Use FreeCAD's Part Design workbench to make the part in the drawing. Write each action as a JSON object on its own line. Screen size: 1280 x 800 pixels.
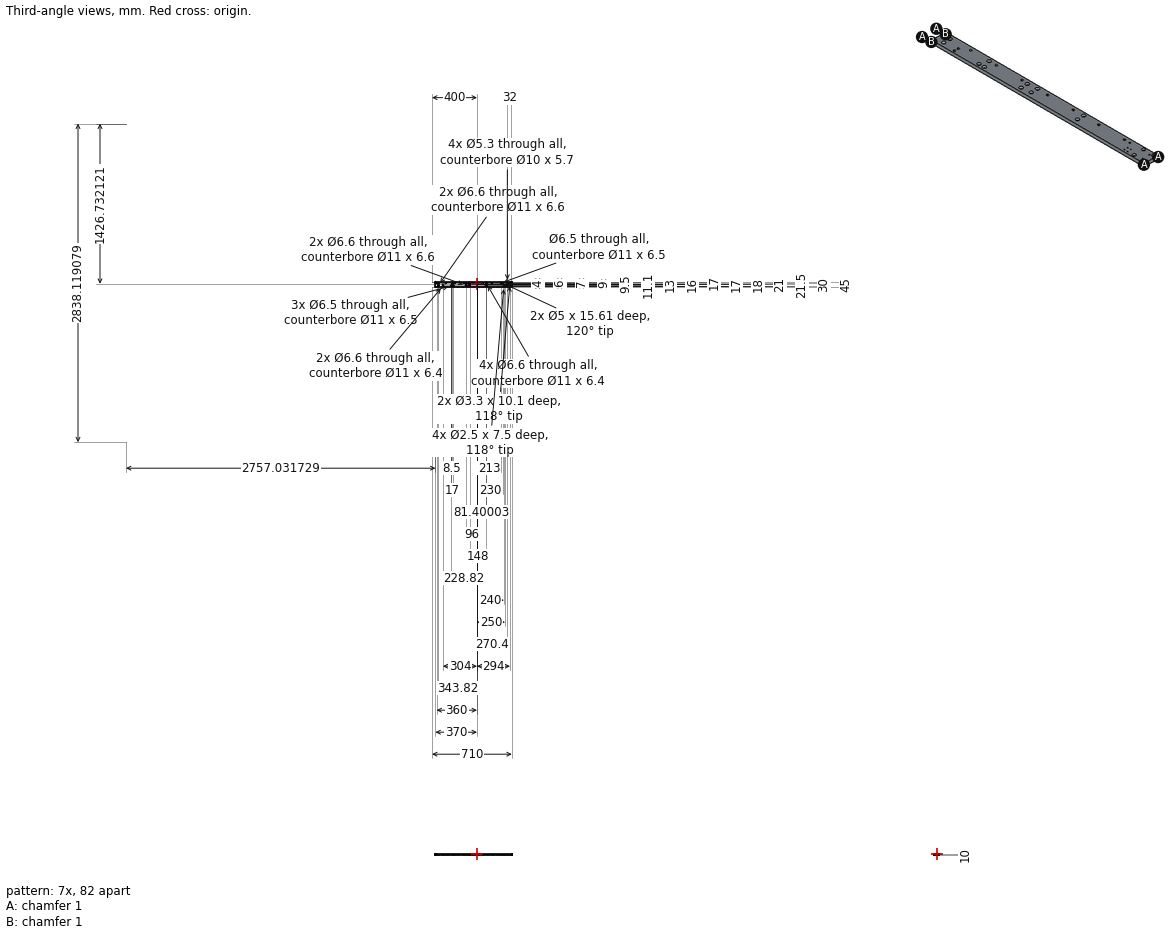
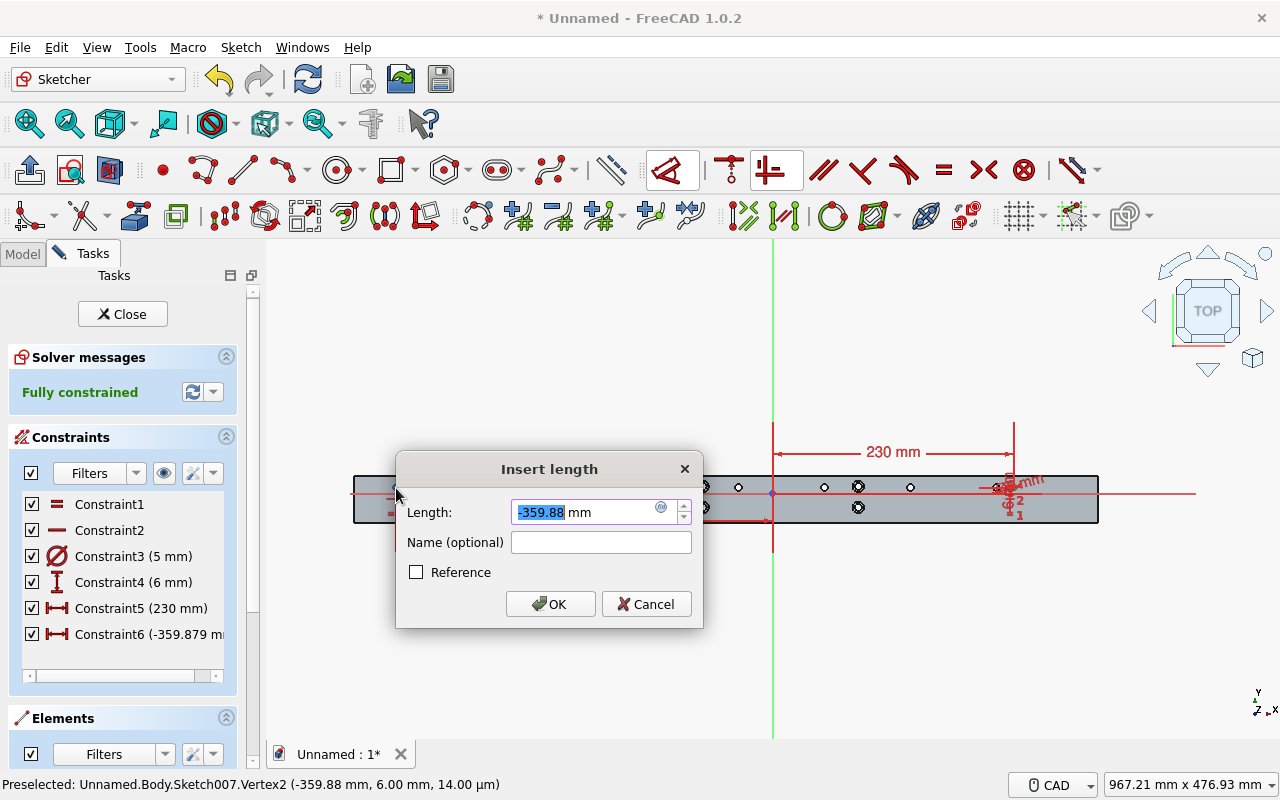
{"action": "type", "text": "-360"}
{"action": "key", "text": "Return"}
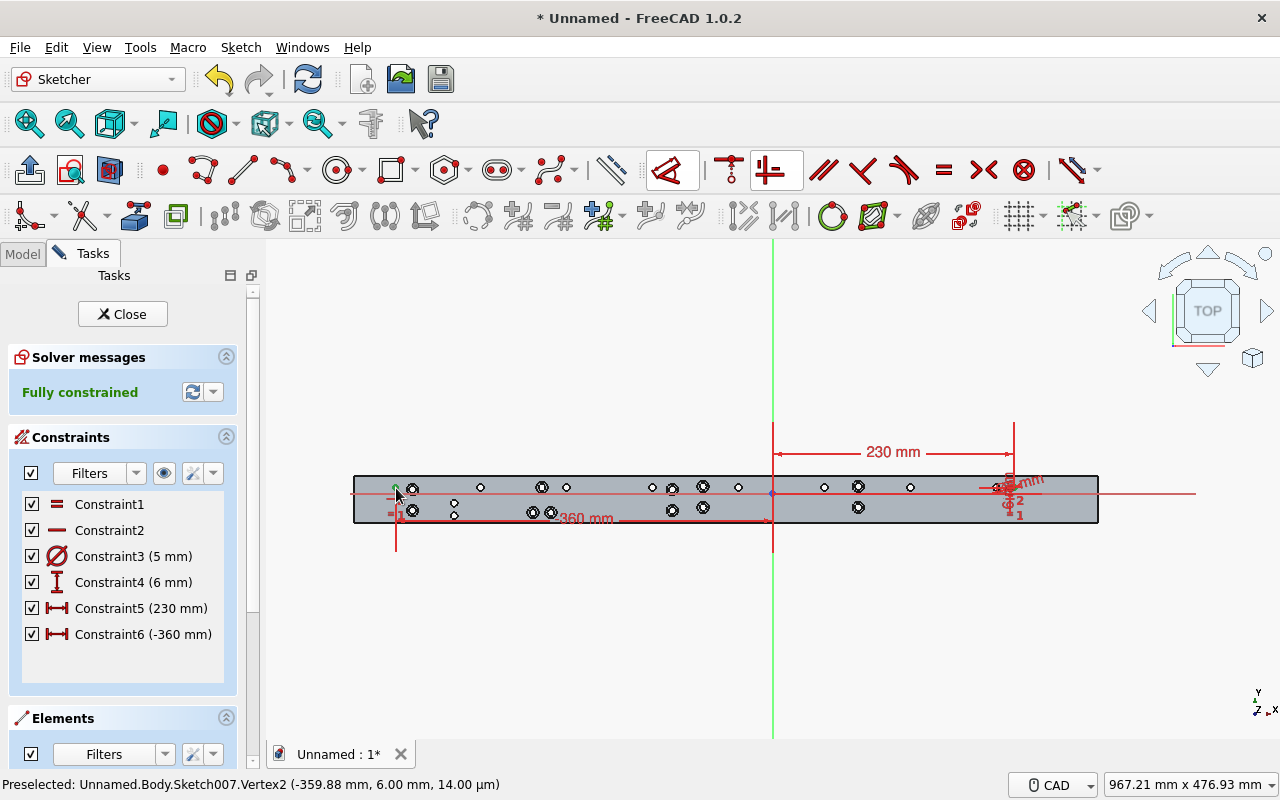
{"action": "left_click", "coordinate": [123, 314]}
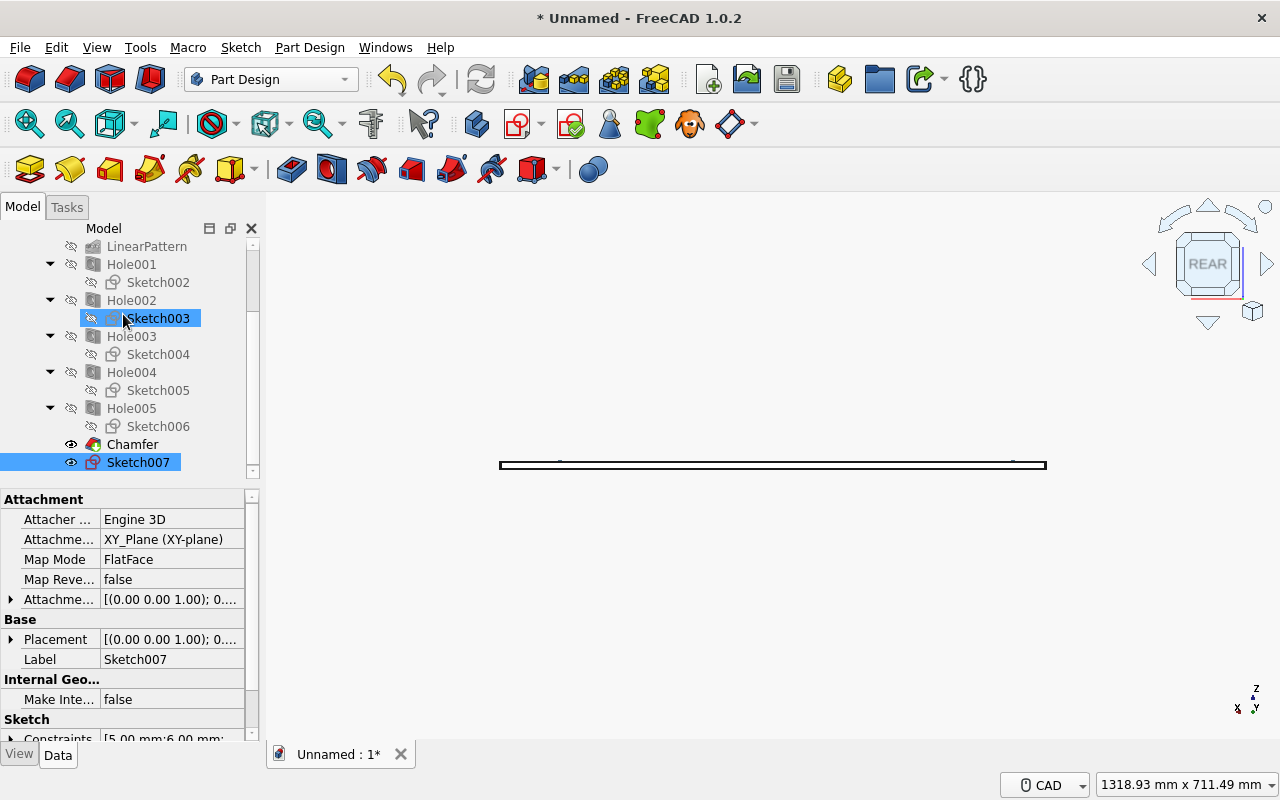
{"action": "left_click", "coordinate": [332, 170]}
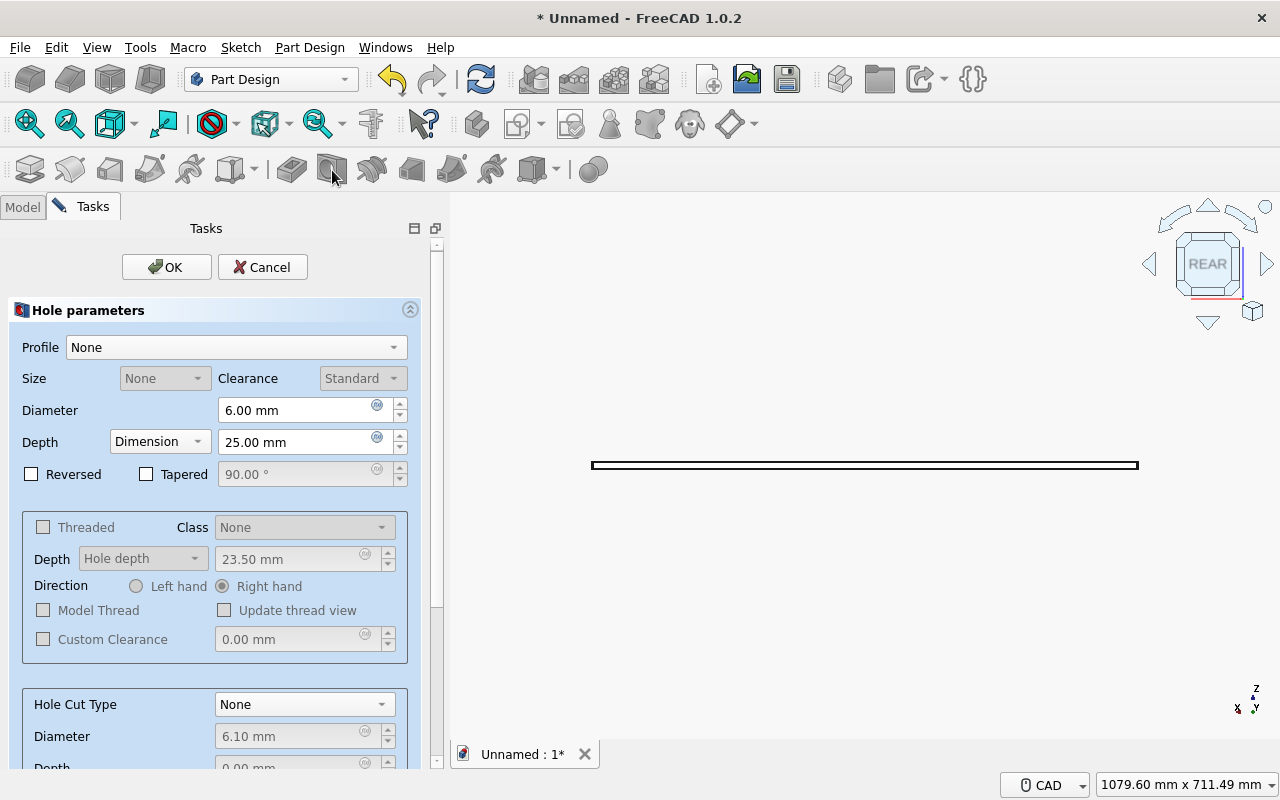
{"action": "triple_click", "coordinate": [305, 410]}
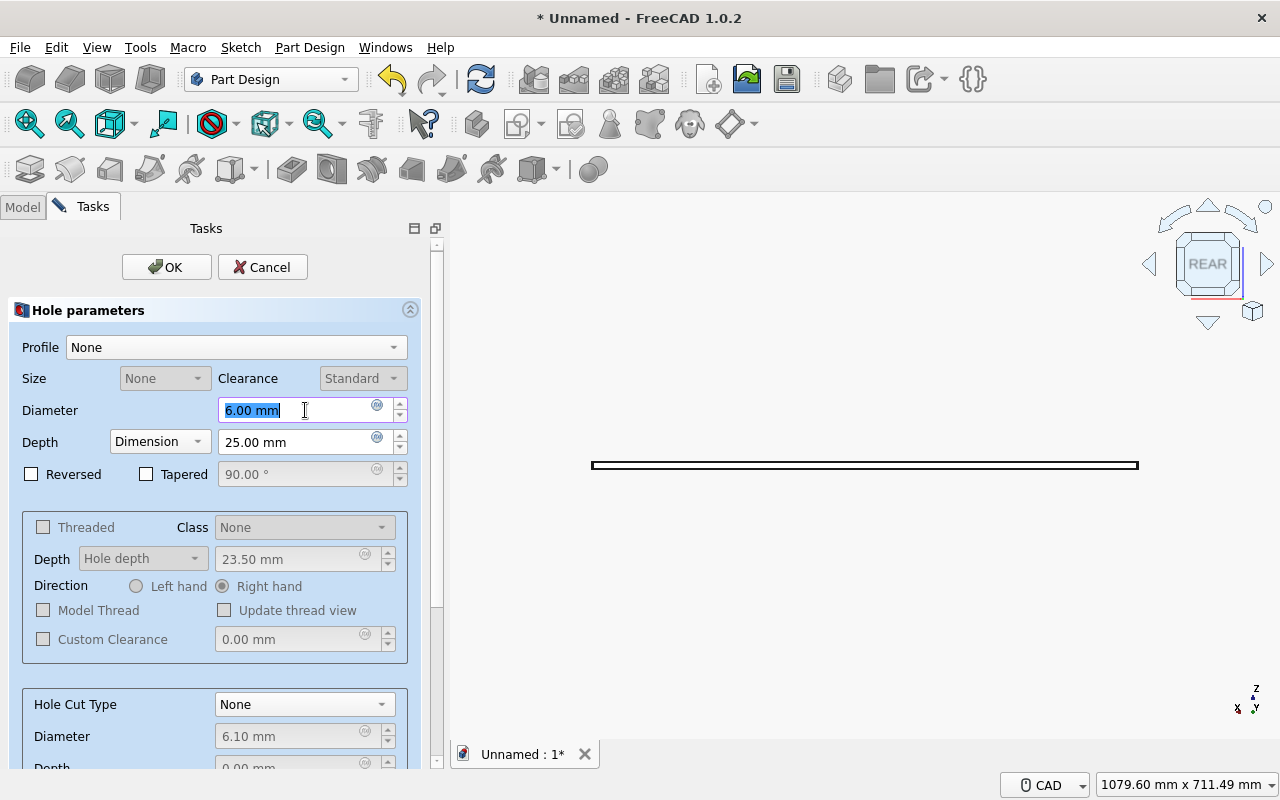
{"action": "type", "text": "5"}
{"action": "key", "text": "Tab"}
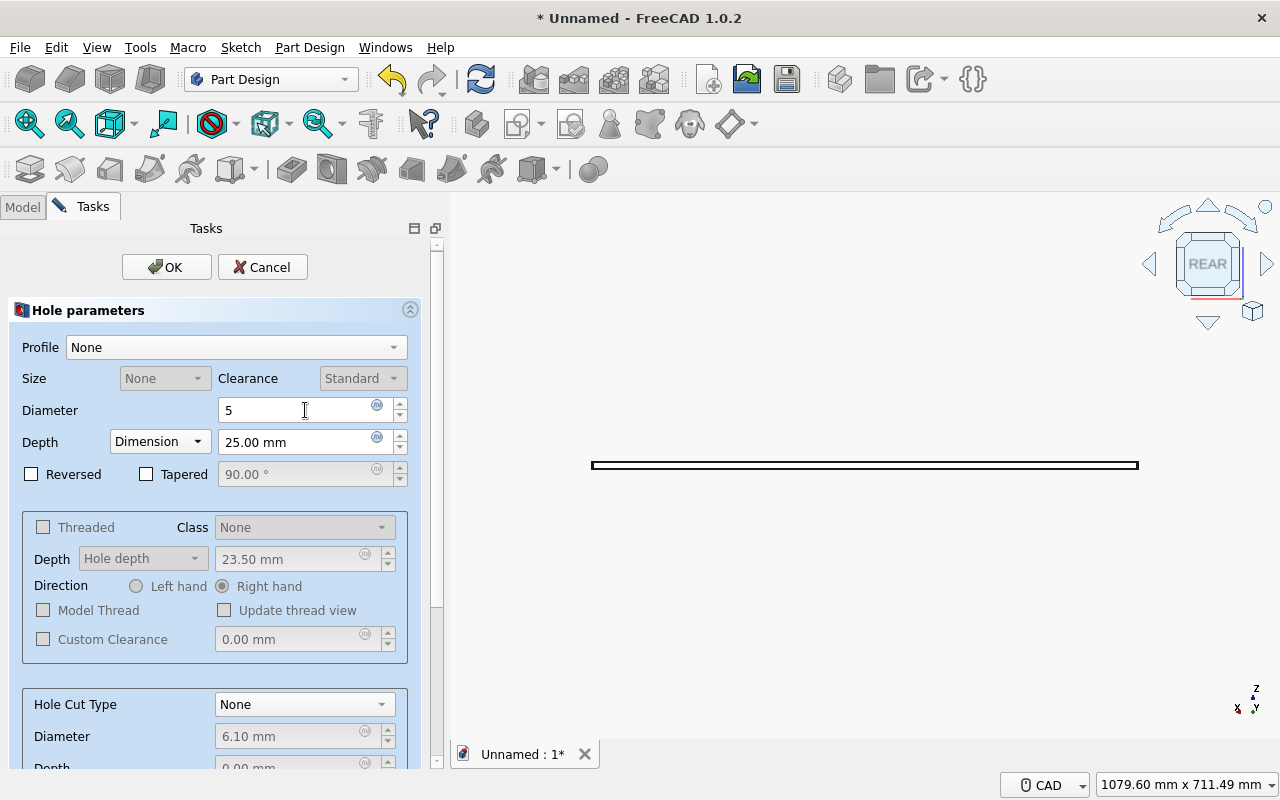
{"action": "triple_click", "coordinate": [305, 442]}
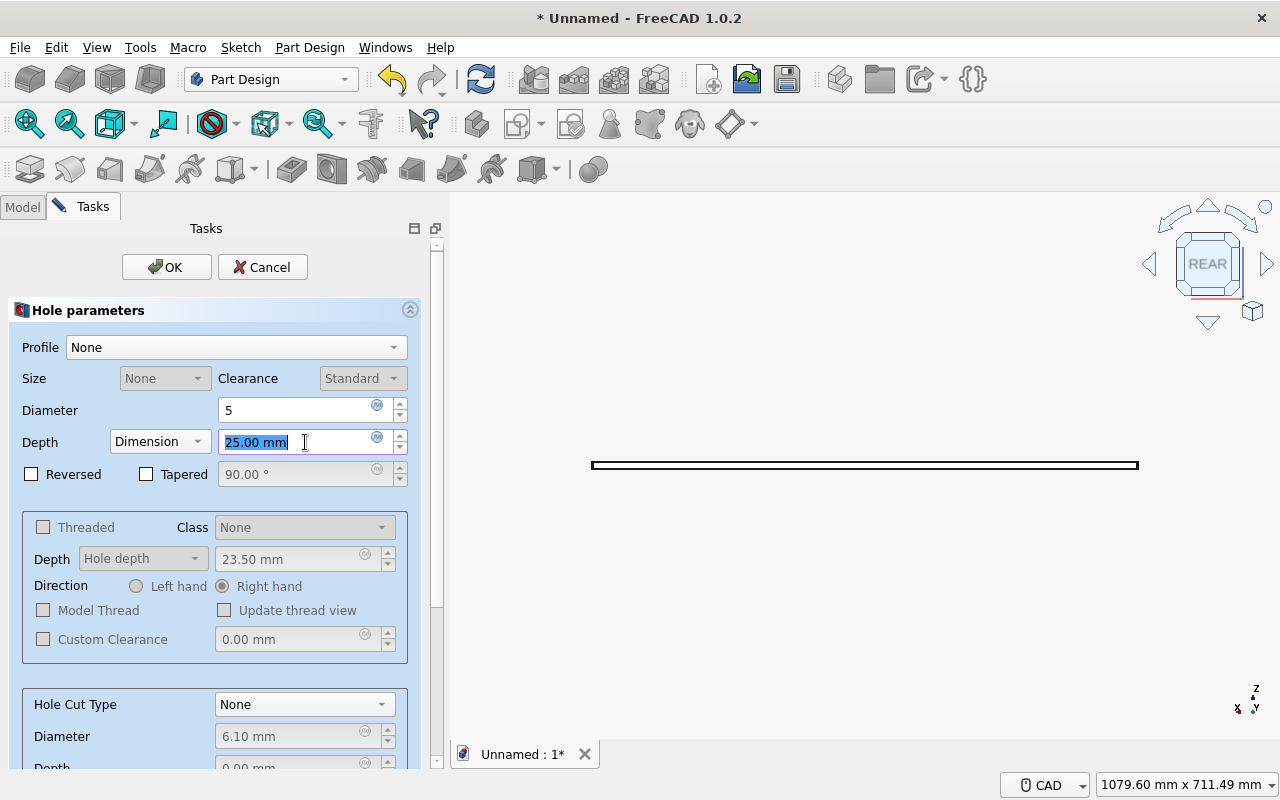
{"action": "type", "text": "15.61"}
{"action": "key", "text": "Tab"}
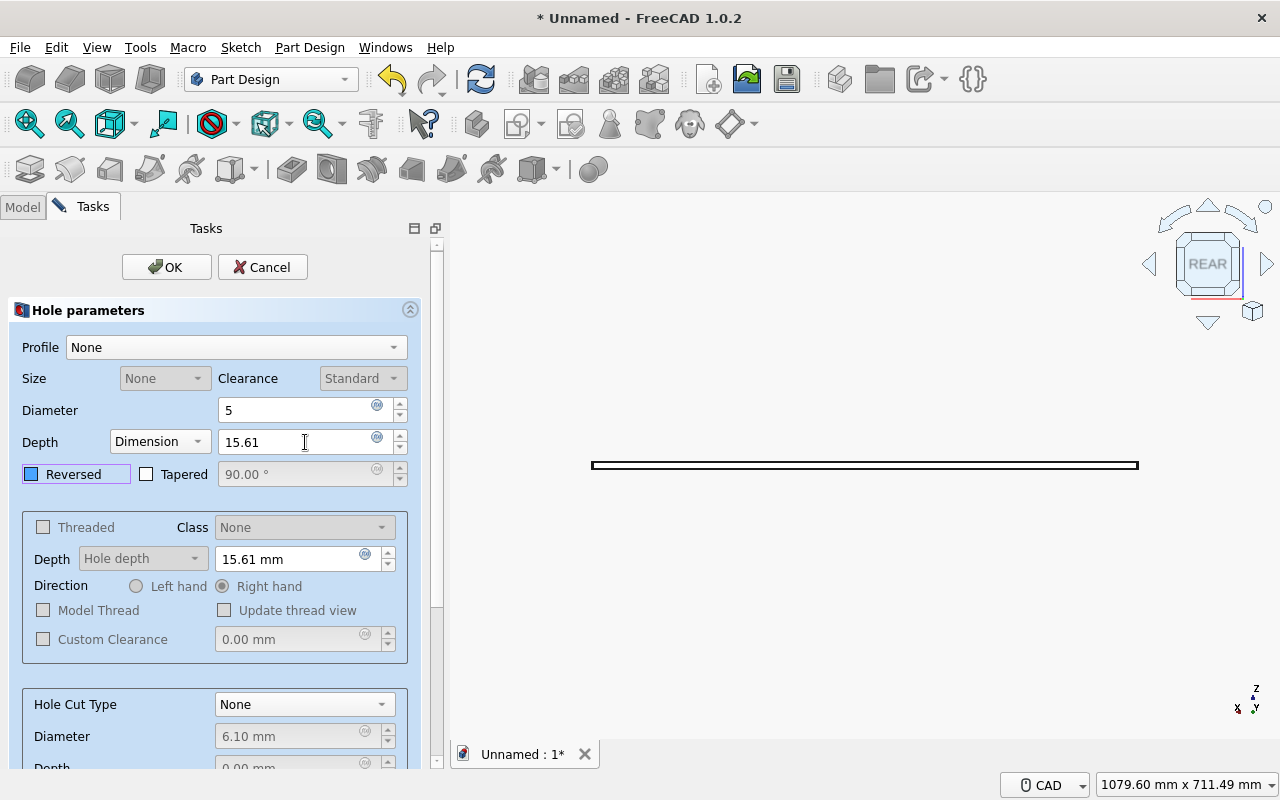
{"action": "scroll", "coordinate": [437, 503], "scroll_direction": "down", "scroll_amount": 4}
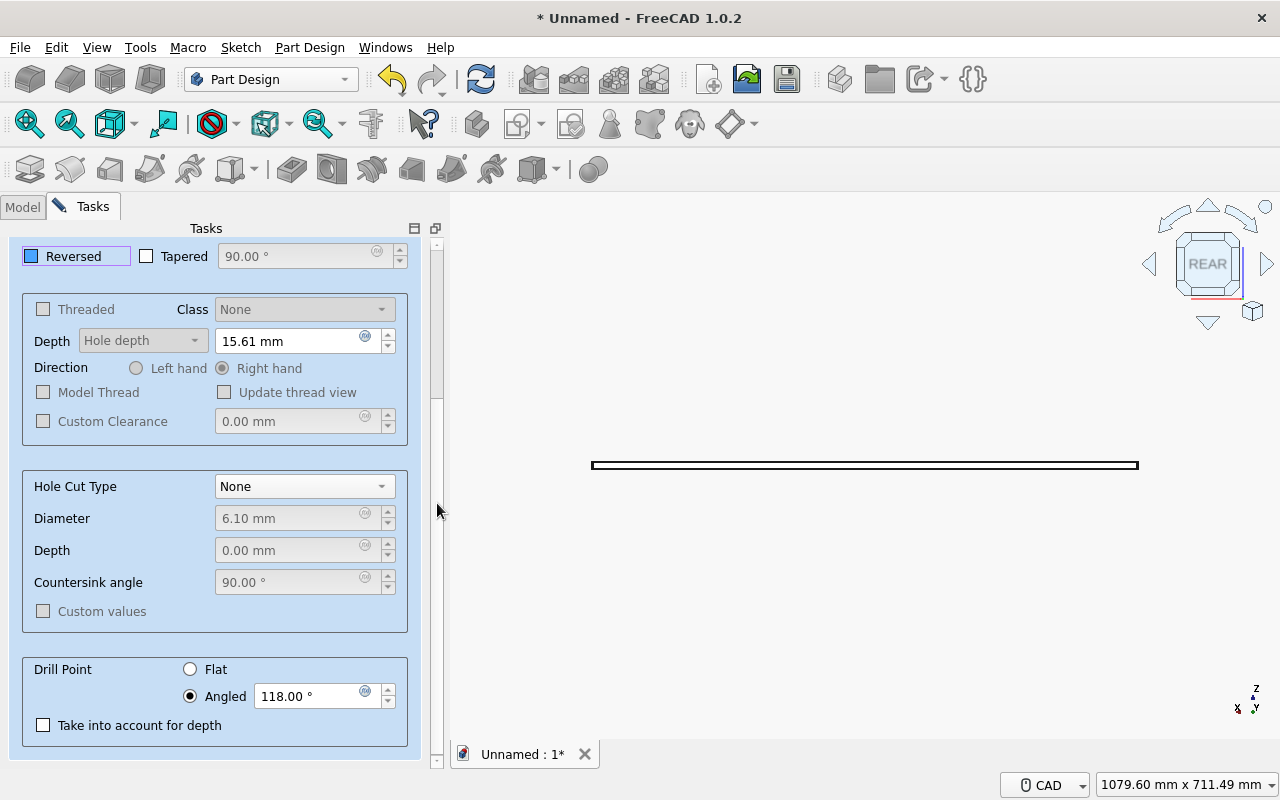
{"action": "triple_click", "coordinate": [317, 696]}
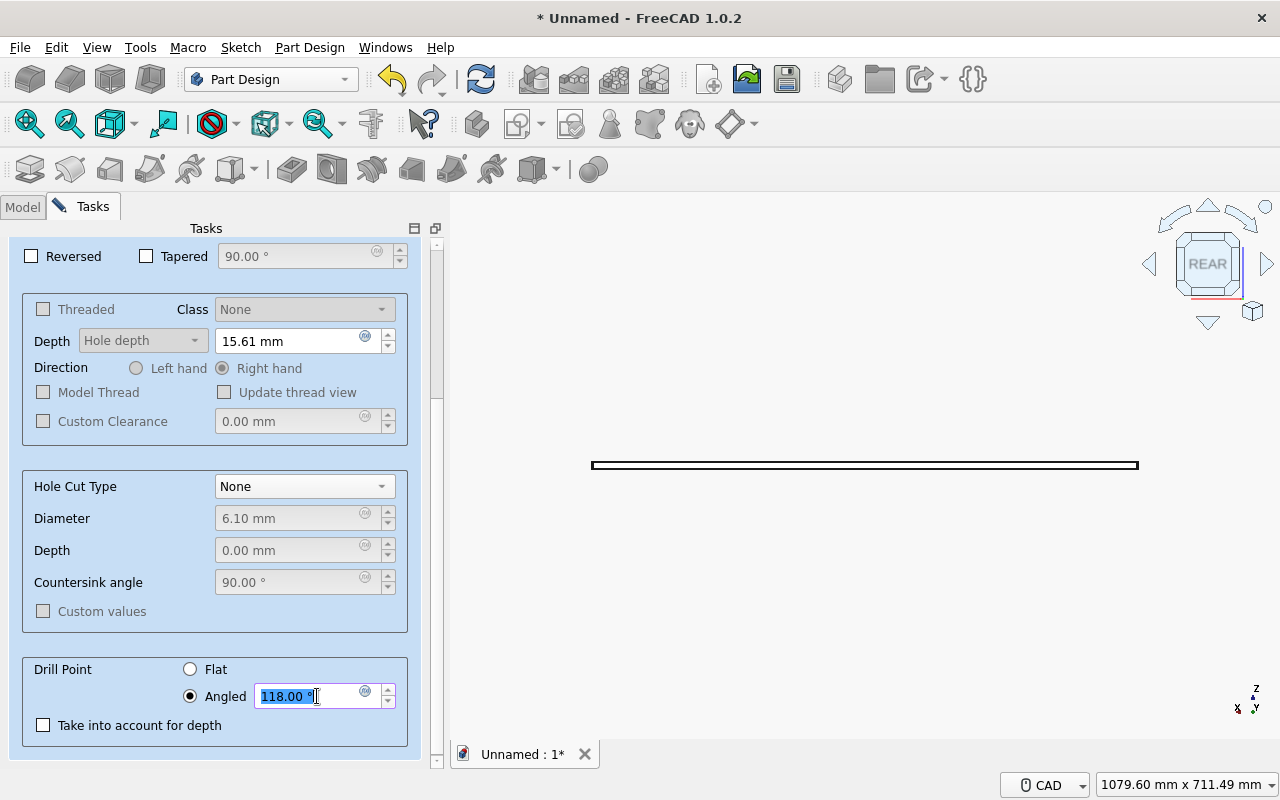
{"action": "type", "text": "120"}
{"action": "key", "text": "Tab"}